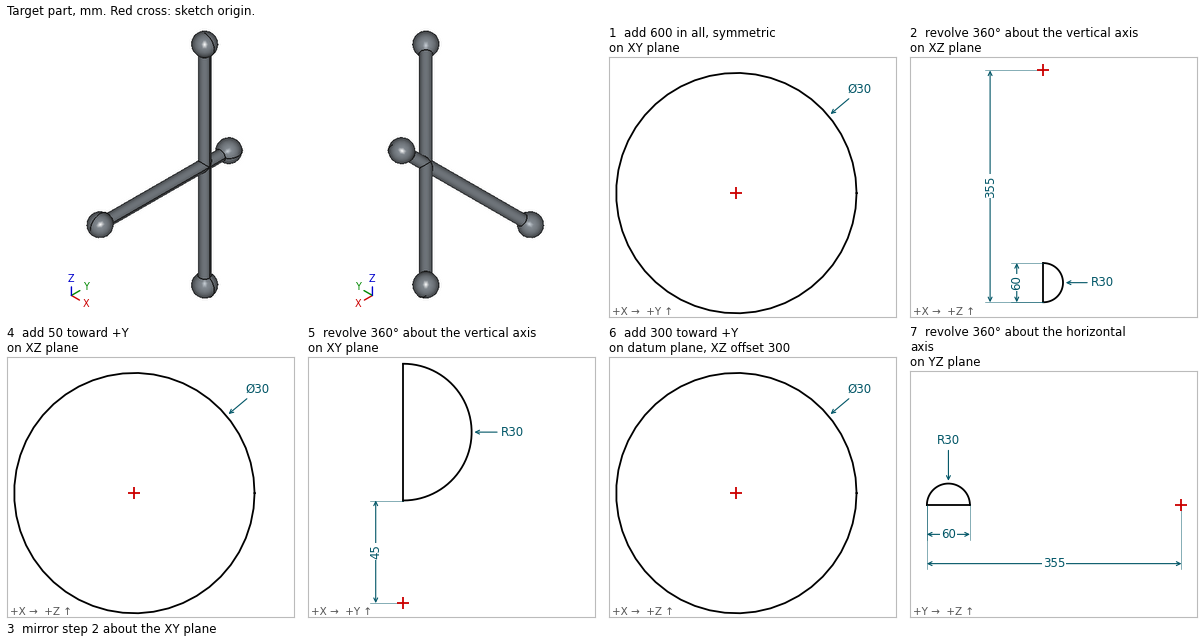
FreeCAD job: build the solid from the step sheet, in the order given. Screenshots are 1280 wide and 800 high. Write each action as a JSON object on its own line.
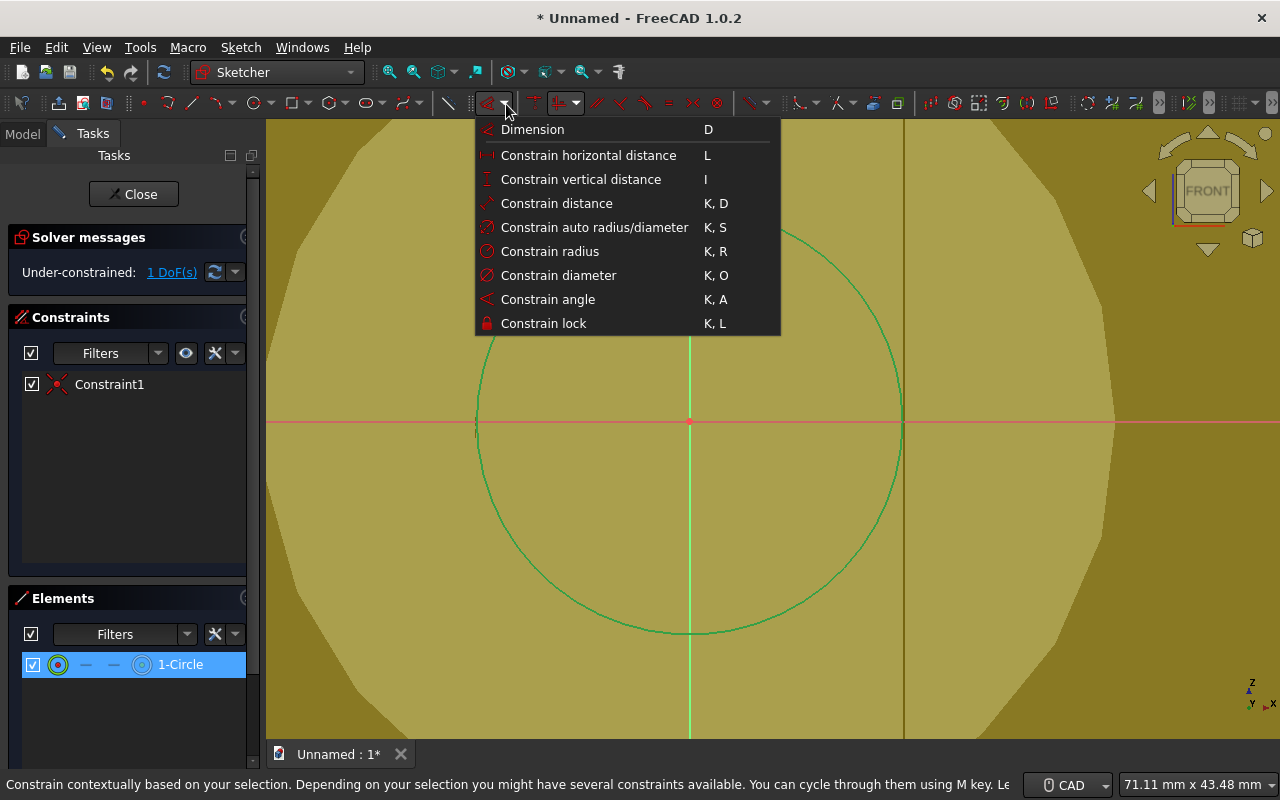
{"action": "left_click", "coordinate": [628, 275]}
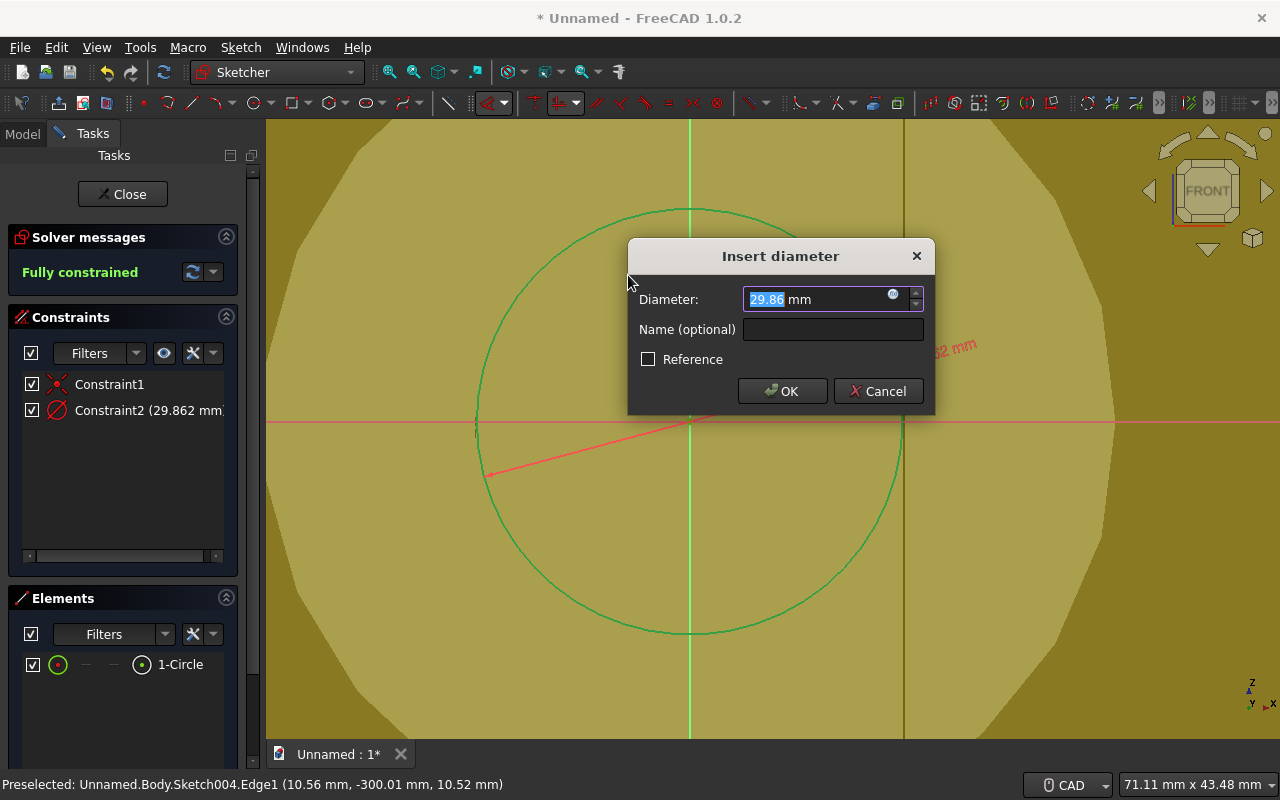
{"action": "type", "text": "30"}
{"action": "key", "text": "Return"}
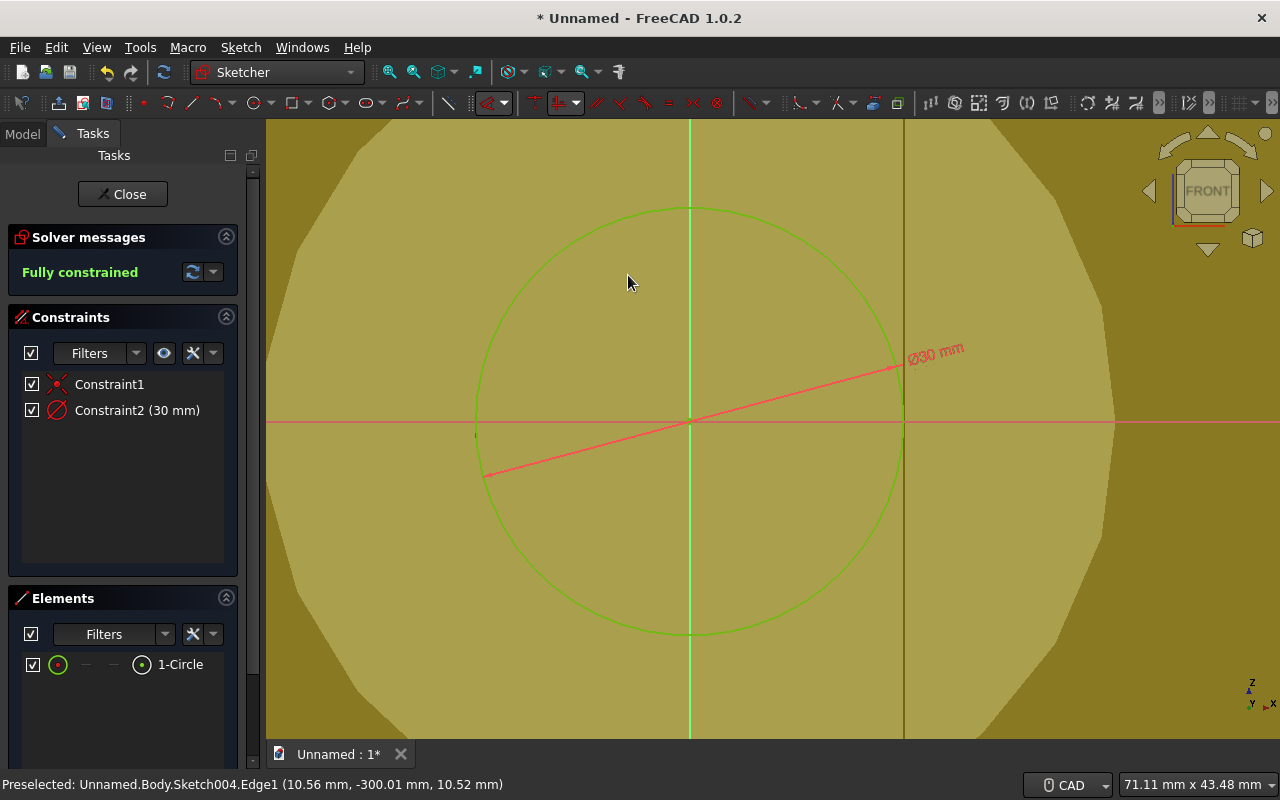
{"action": "left_click", "coordinate": [123, 194]}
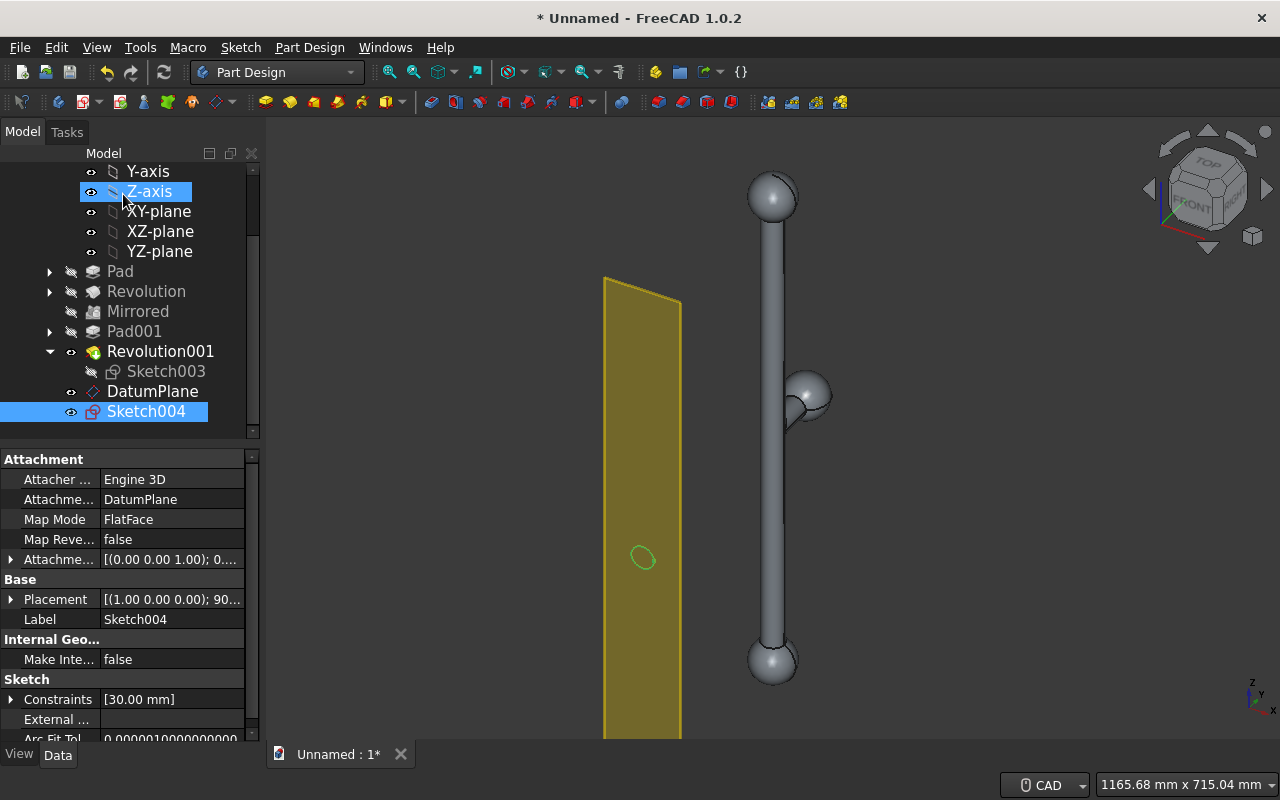
{"action": "left_click", "coordinate": [266, 102]}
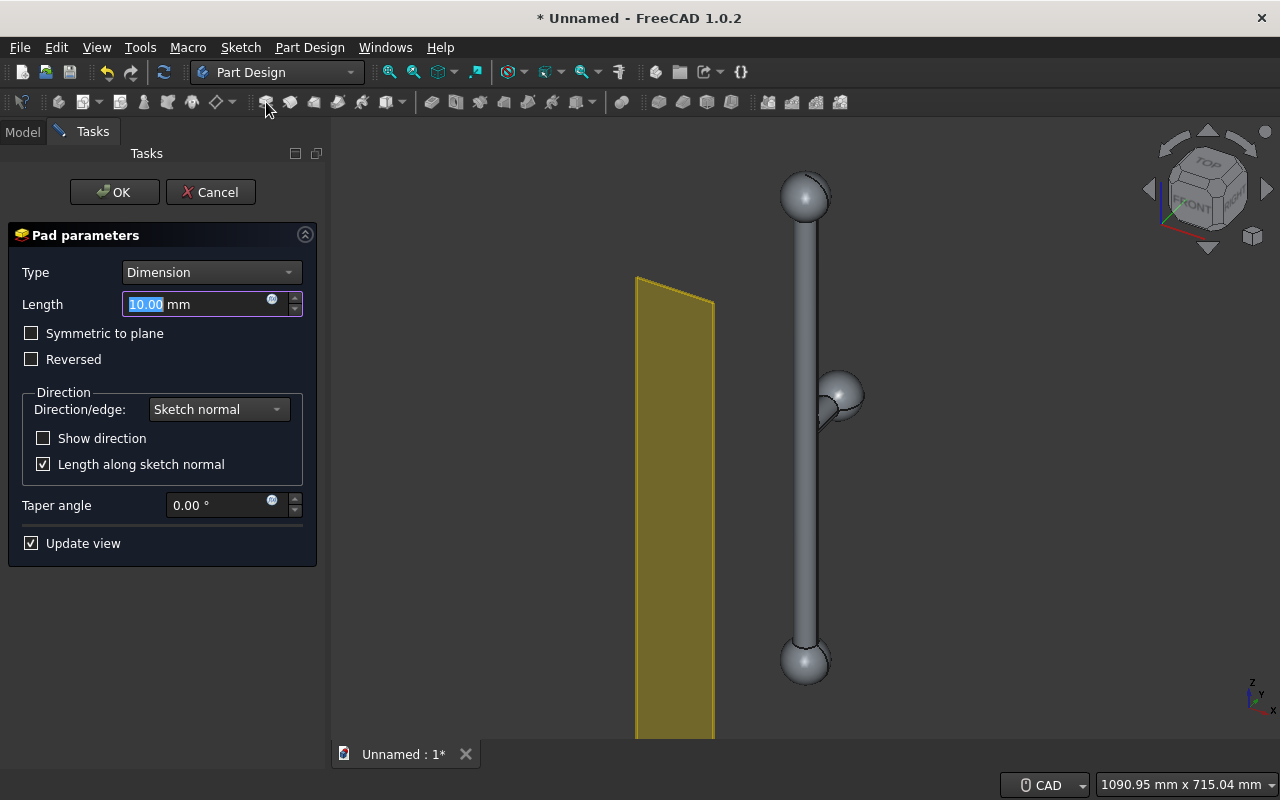
{"action": "type", "text": "300"}
{"action": "key", "text": "Tab"}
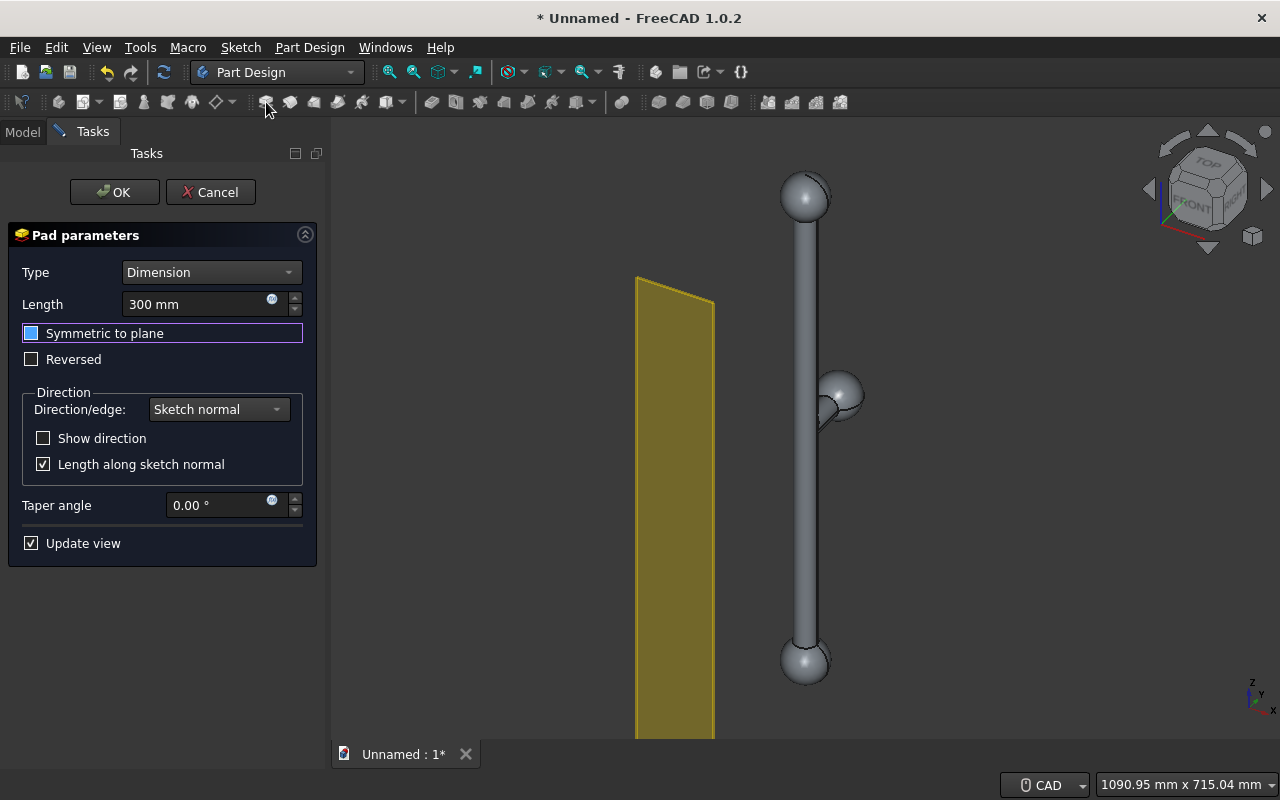
{"action": "left_click", "coordinate": [30, 359]}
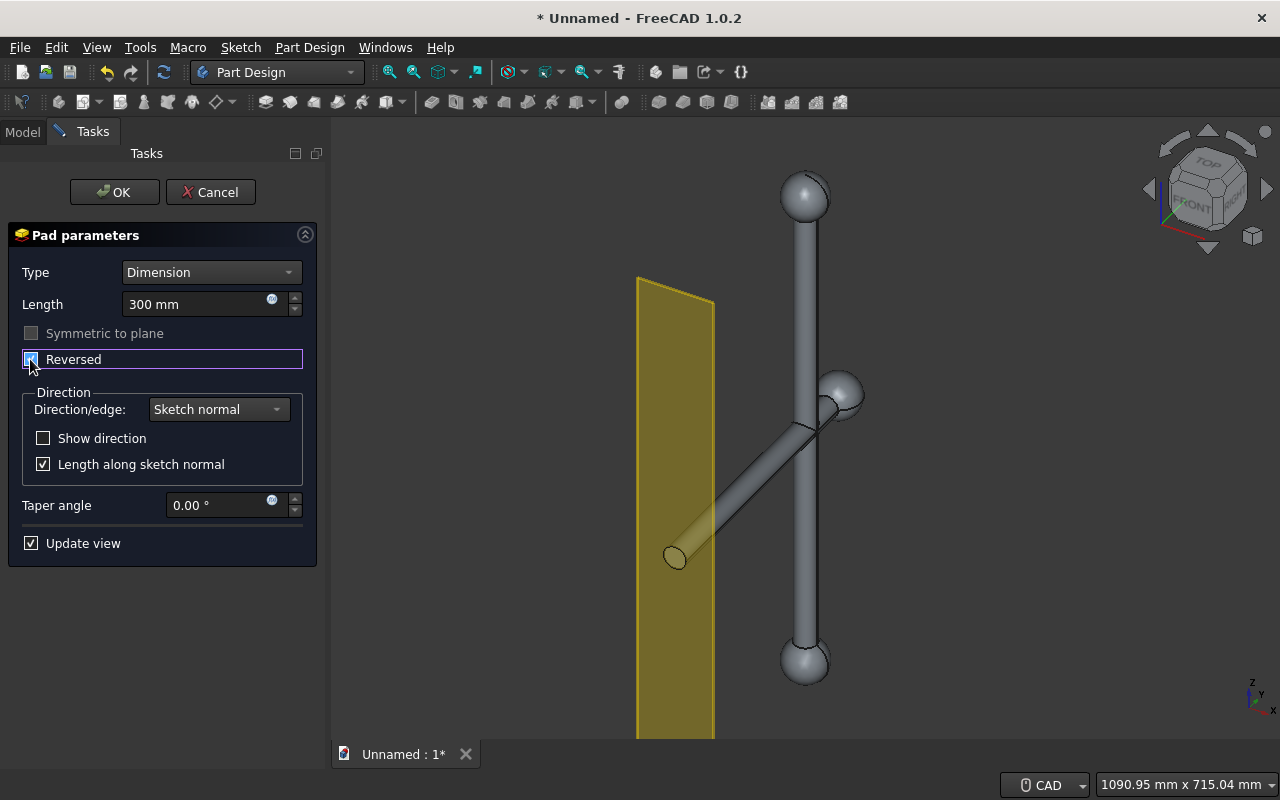
{"action": "left_click", "coordinate": [115, 192]}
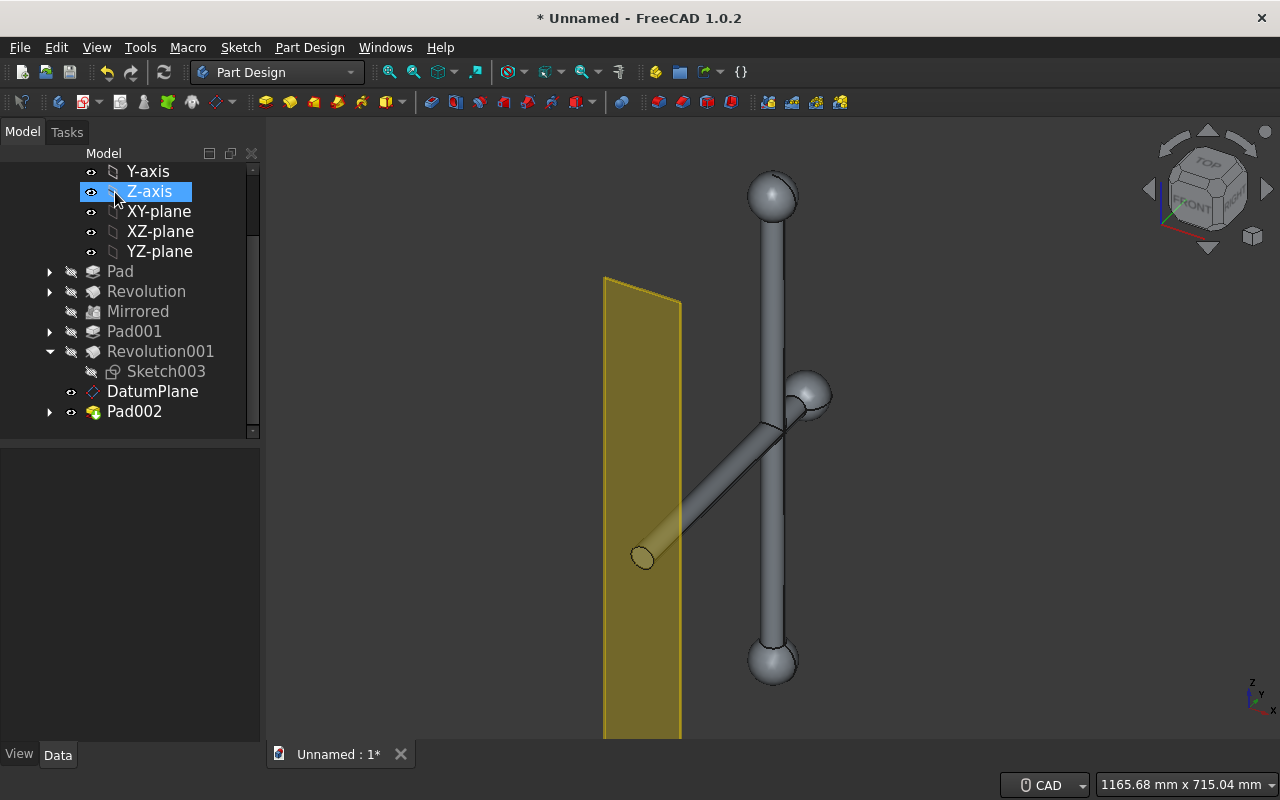
{"action": "left_click", "coordinate": [116, 392]}
{"action": "key", "text": "space"}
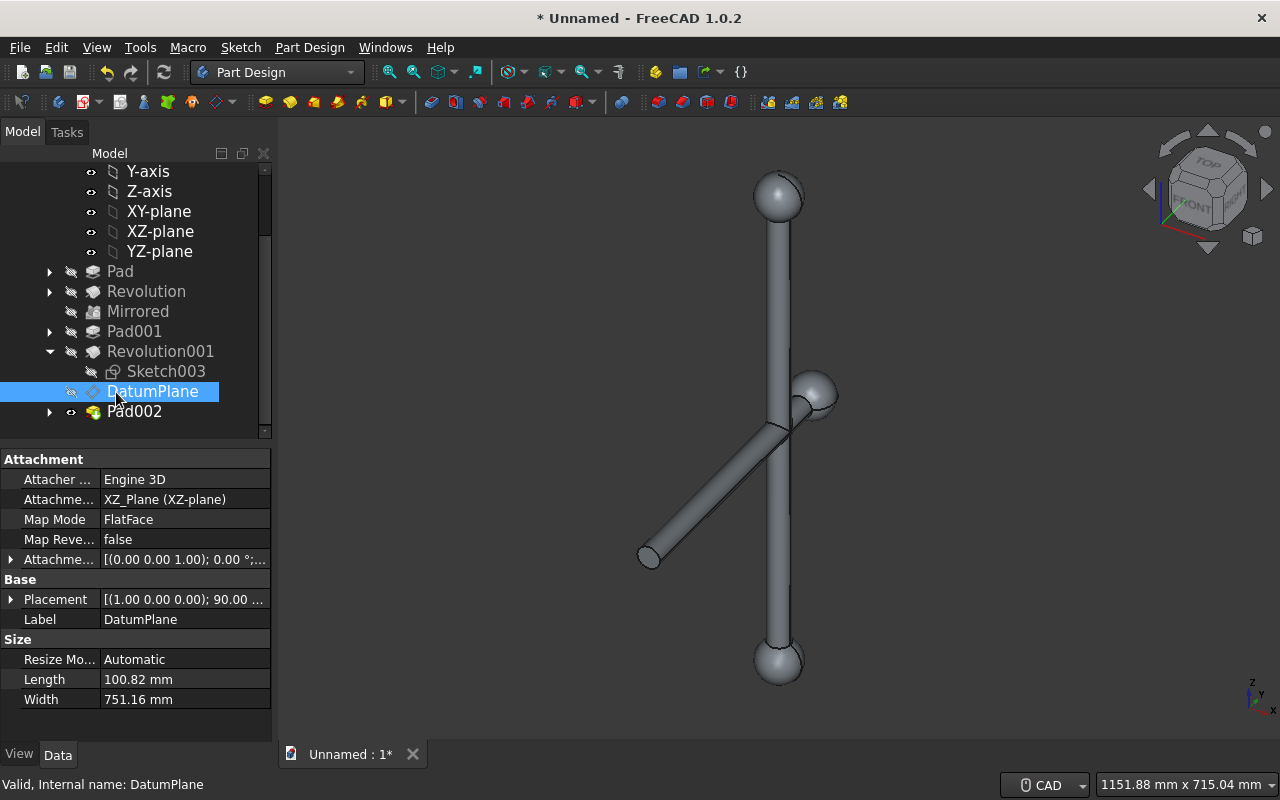
{"action": "left_click", "coordinate": [390, 72]}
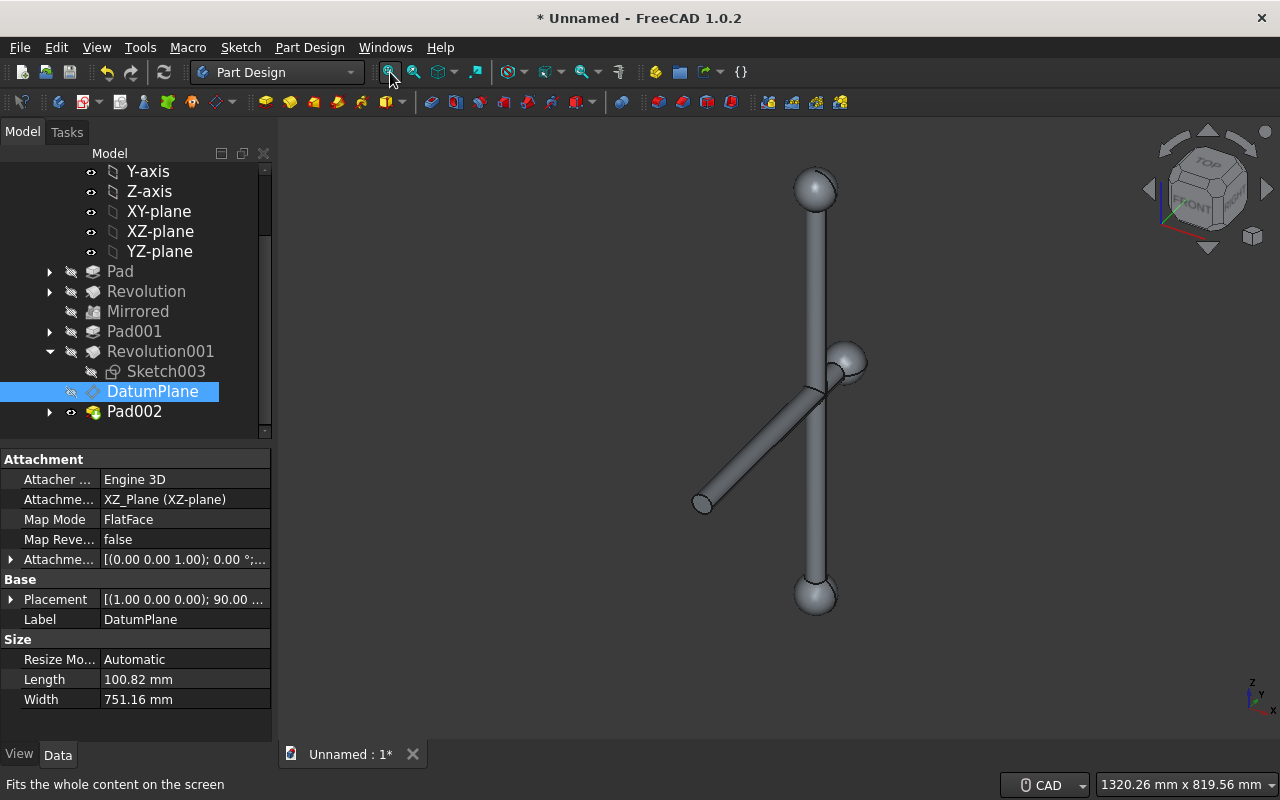
{"action": "left_click", "coordinate": [318, 699]}